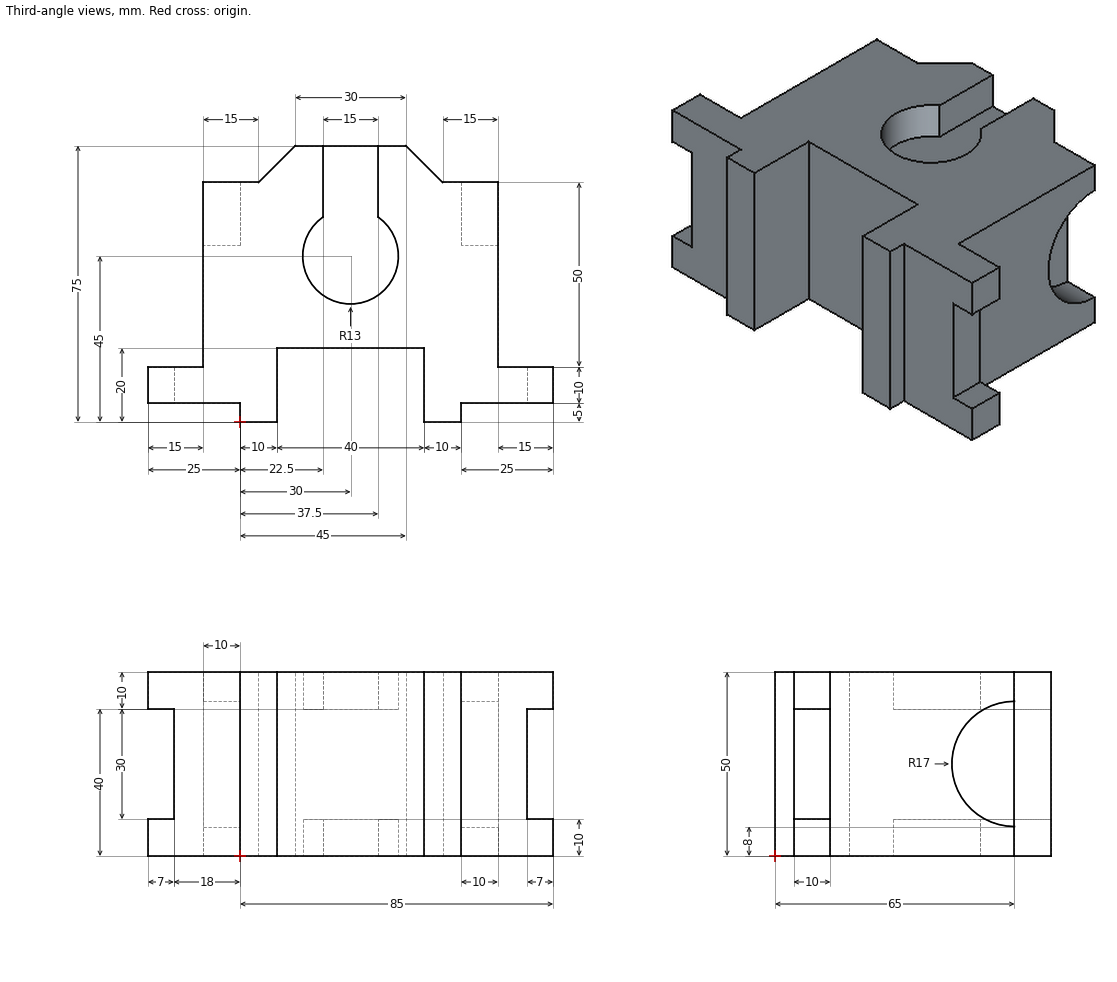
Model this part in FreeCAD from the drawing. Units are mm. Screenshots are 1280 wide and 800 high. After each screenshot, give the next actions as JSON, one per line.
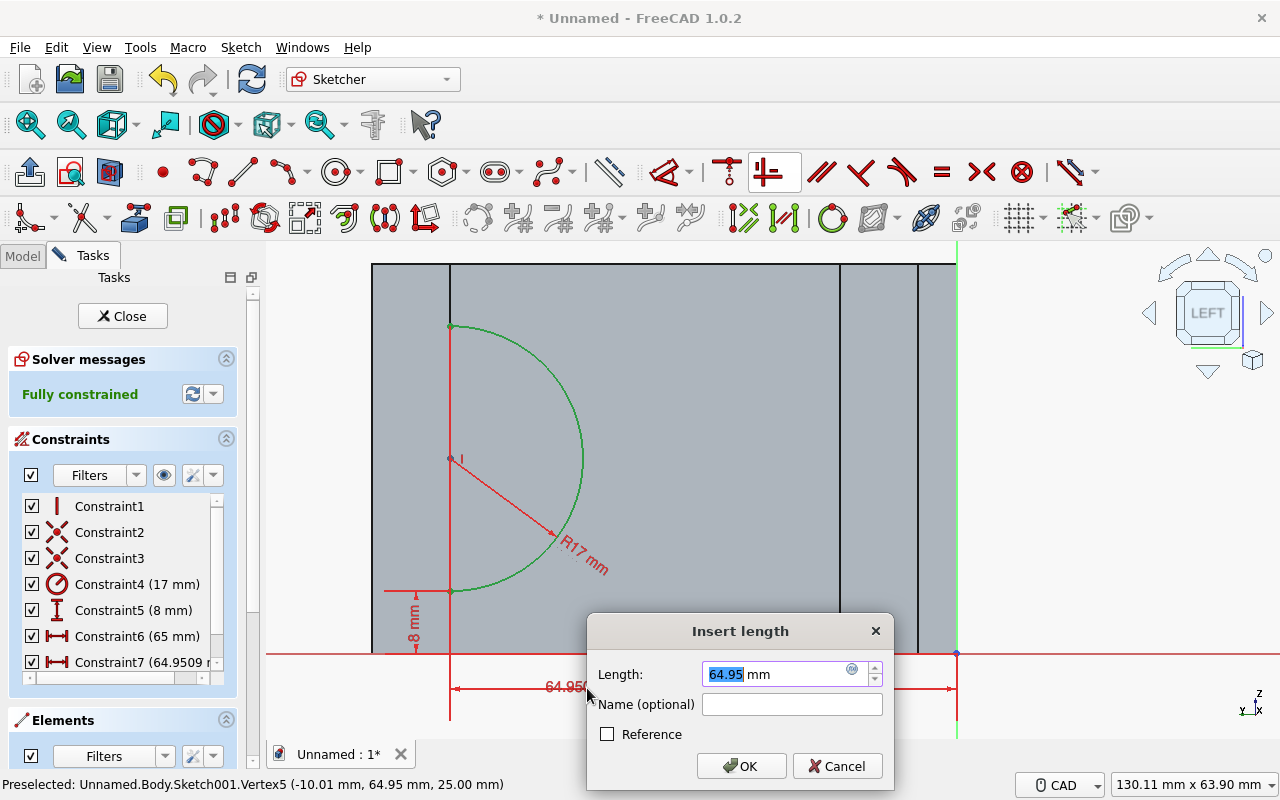
{"action": "type", "text": "65"}
{"action": "key", "text": "Return"}
{"action": "key", "text": "Escape"}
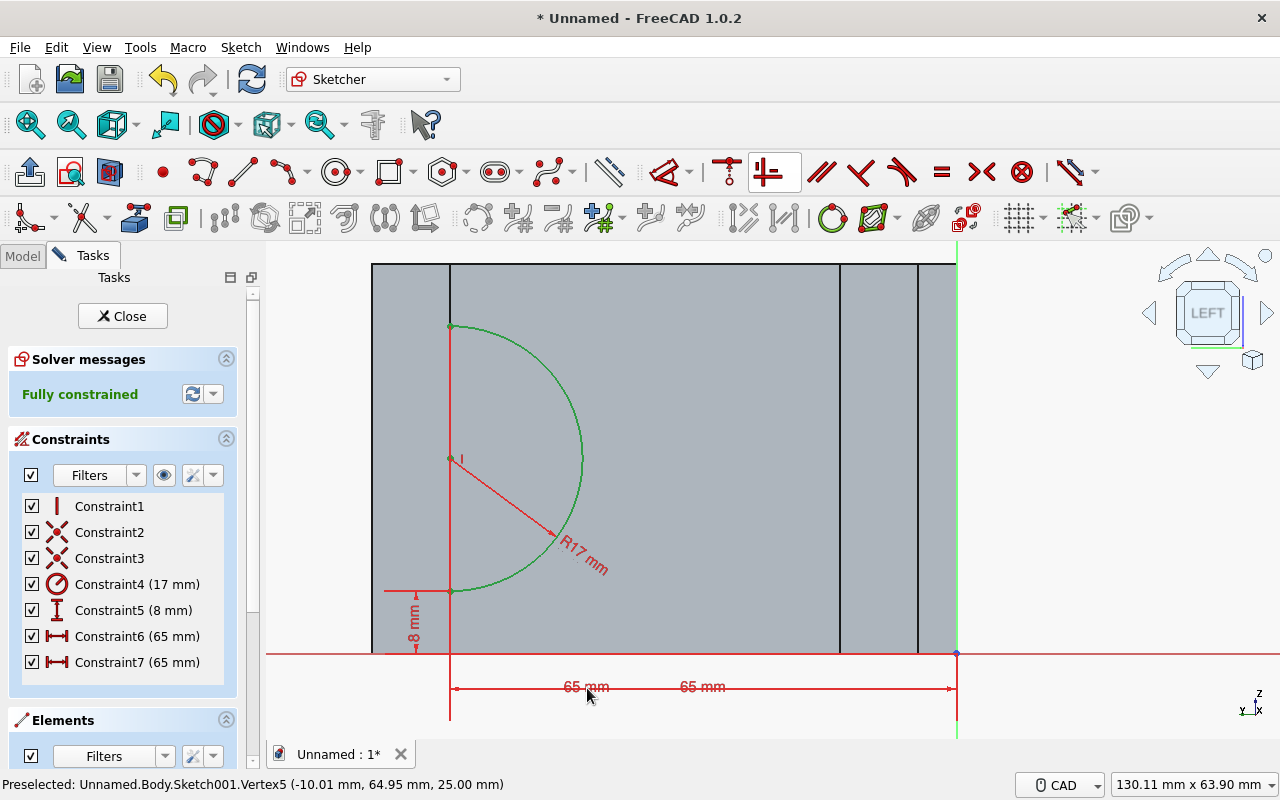
{"action": "left_click", "coordinate": [123, 316]}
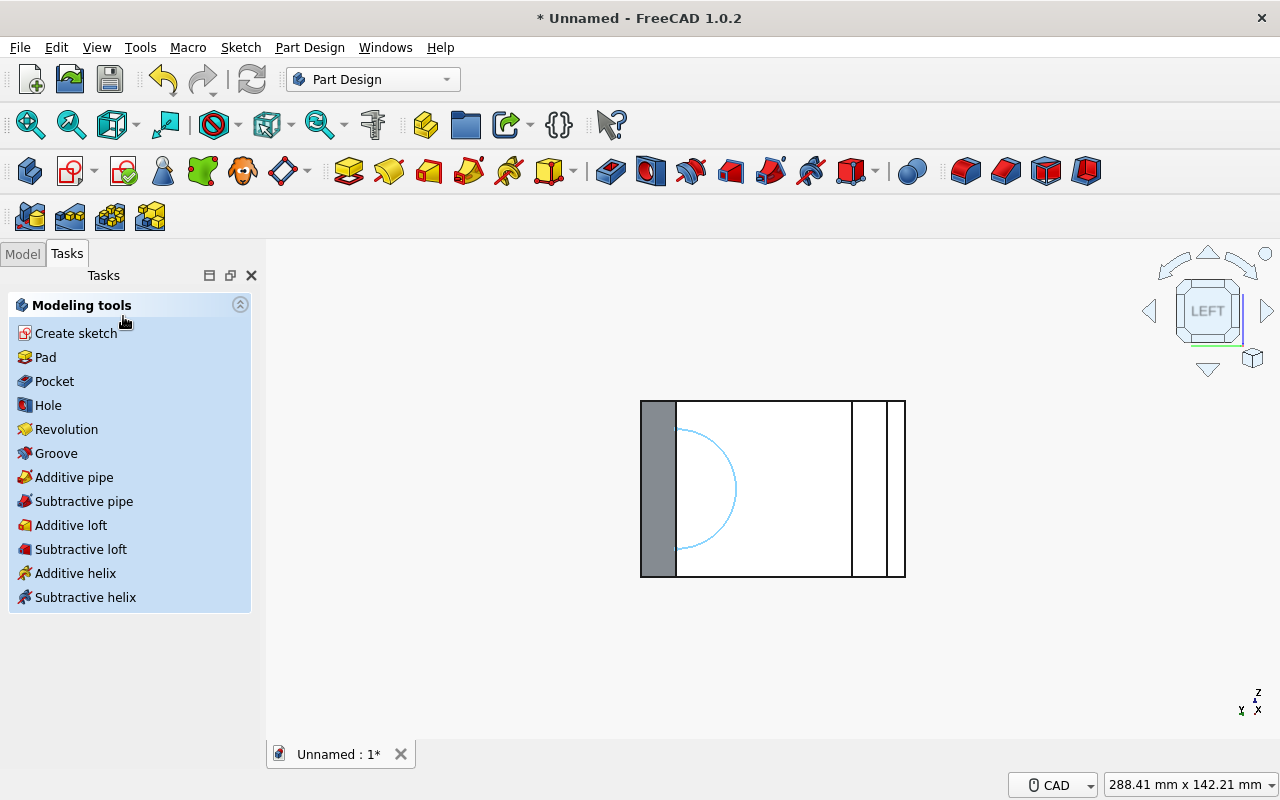
{"action": "left_click", "coordinate": [612, 172]}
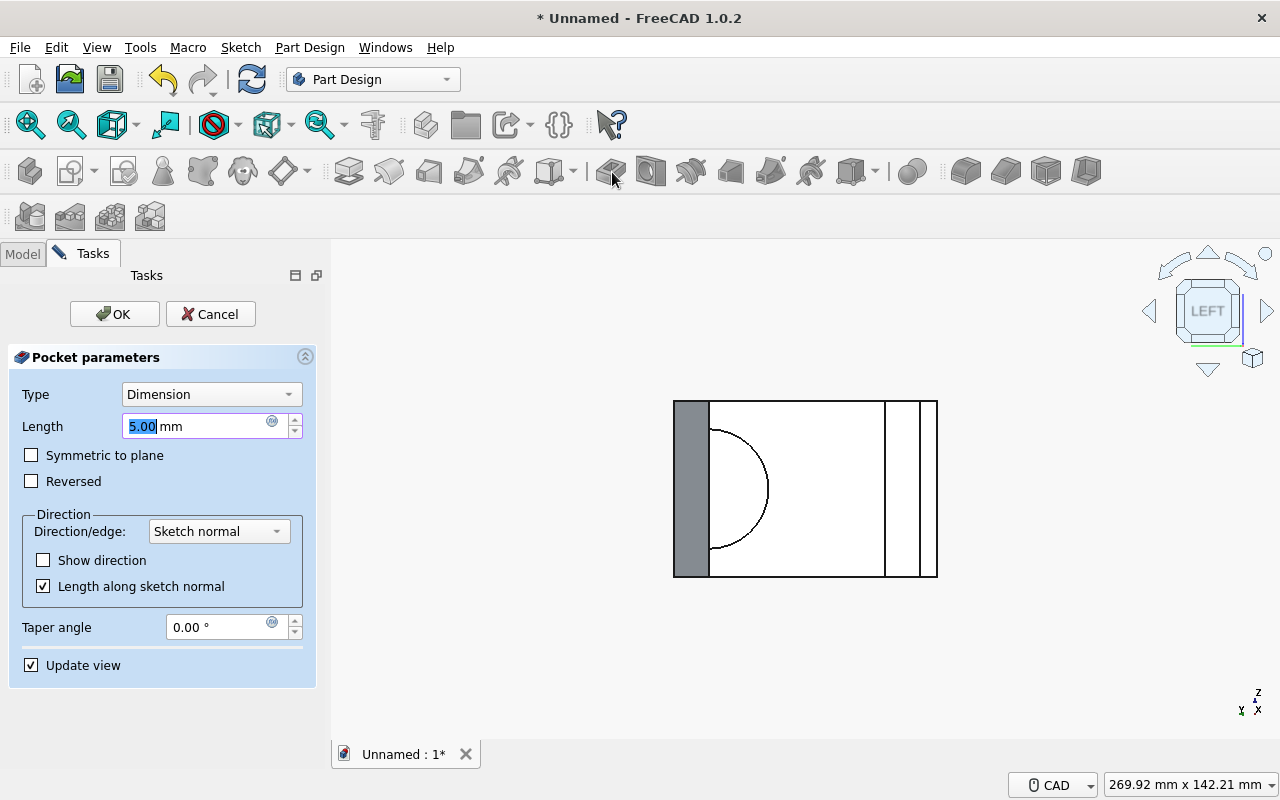
{"action": "type", "text": "10"}
{"action": "key", "text": "Tab"}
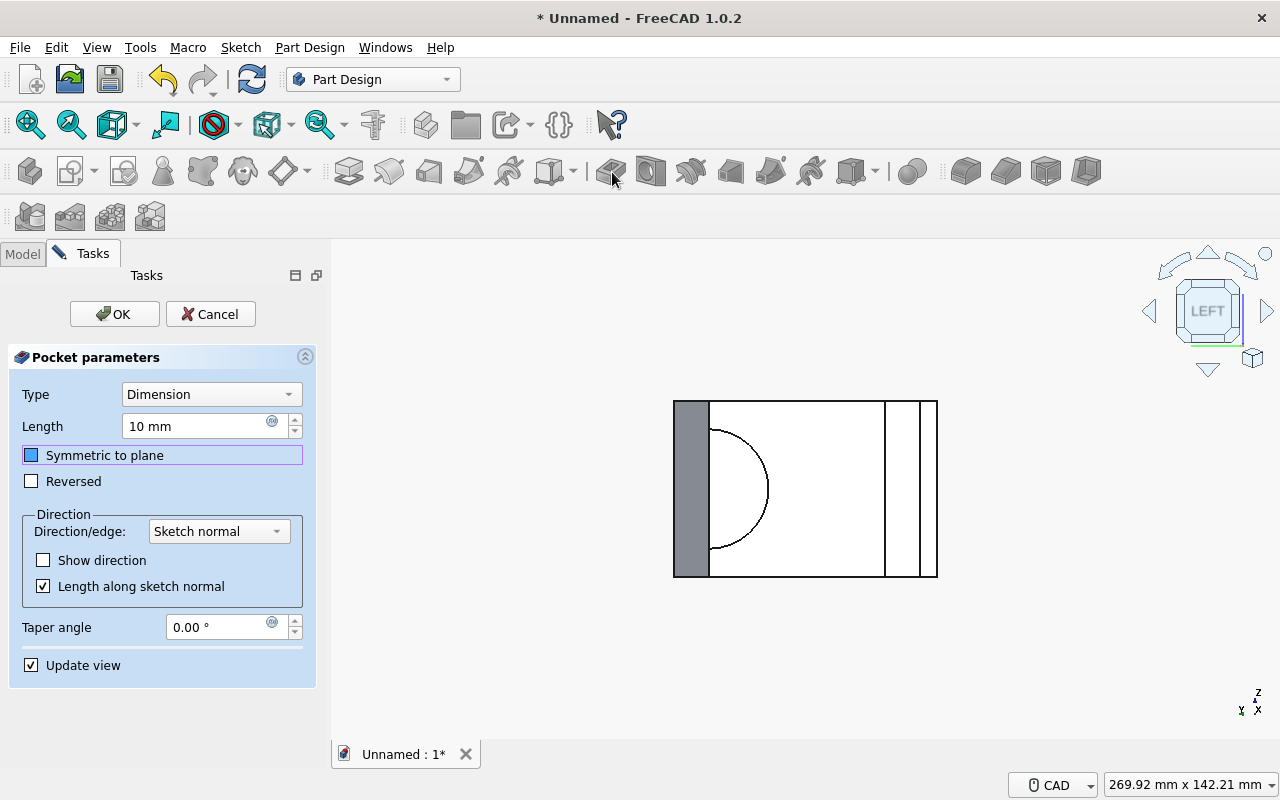
{"action": "left_click", "coordinate": [115, 314]}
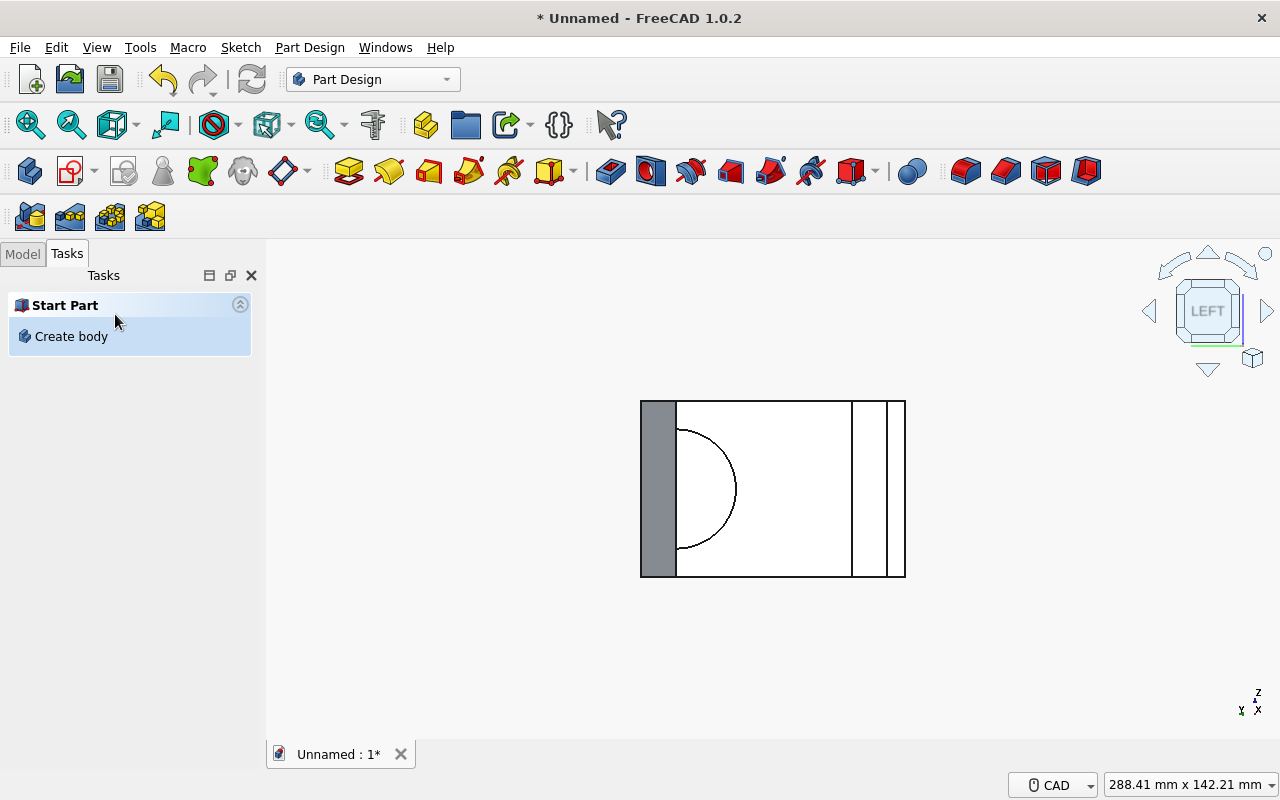
{"action": "left_click", "coordinate": [32, 126]}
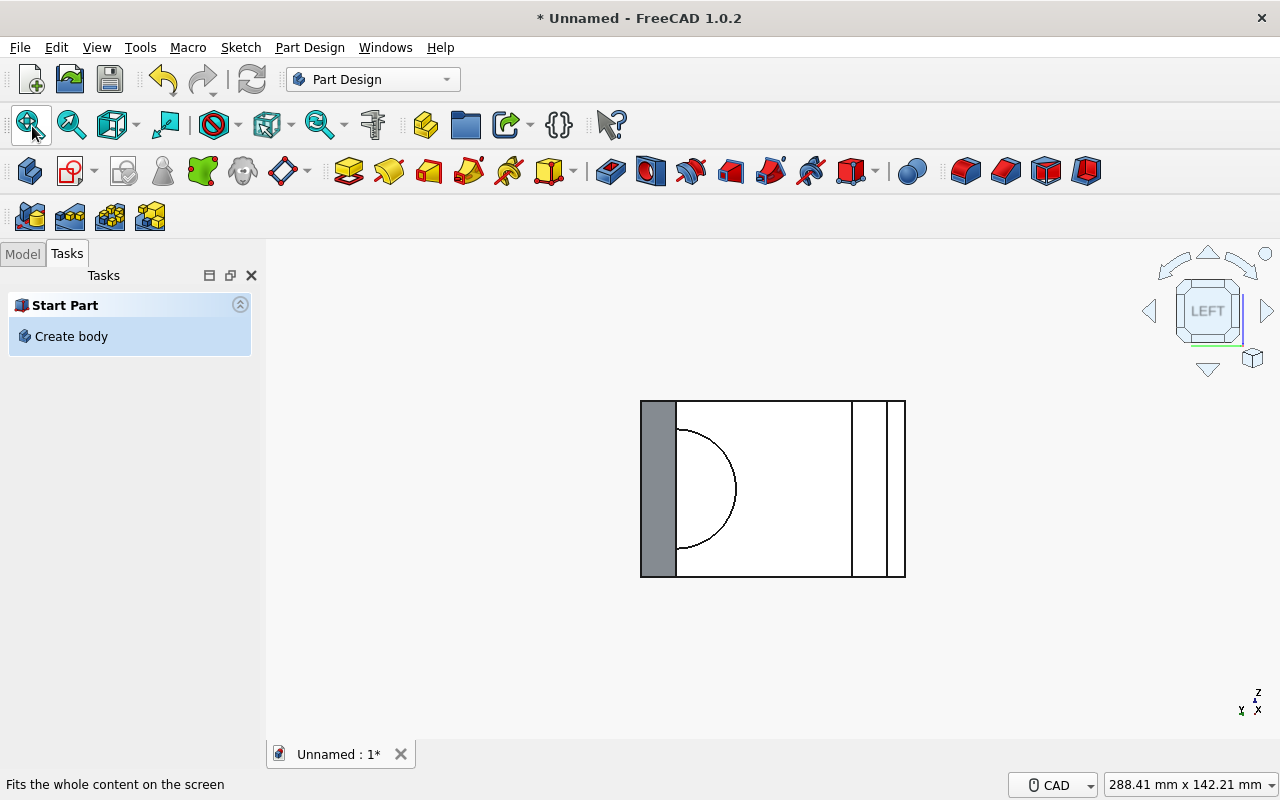
{"action": "key", "text": "0"}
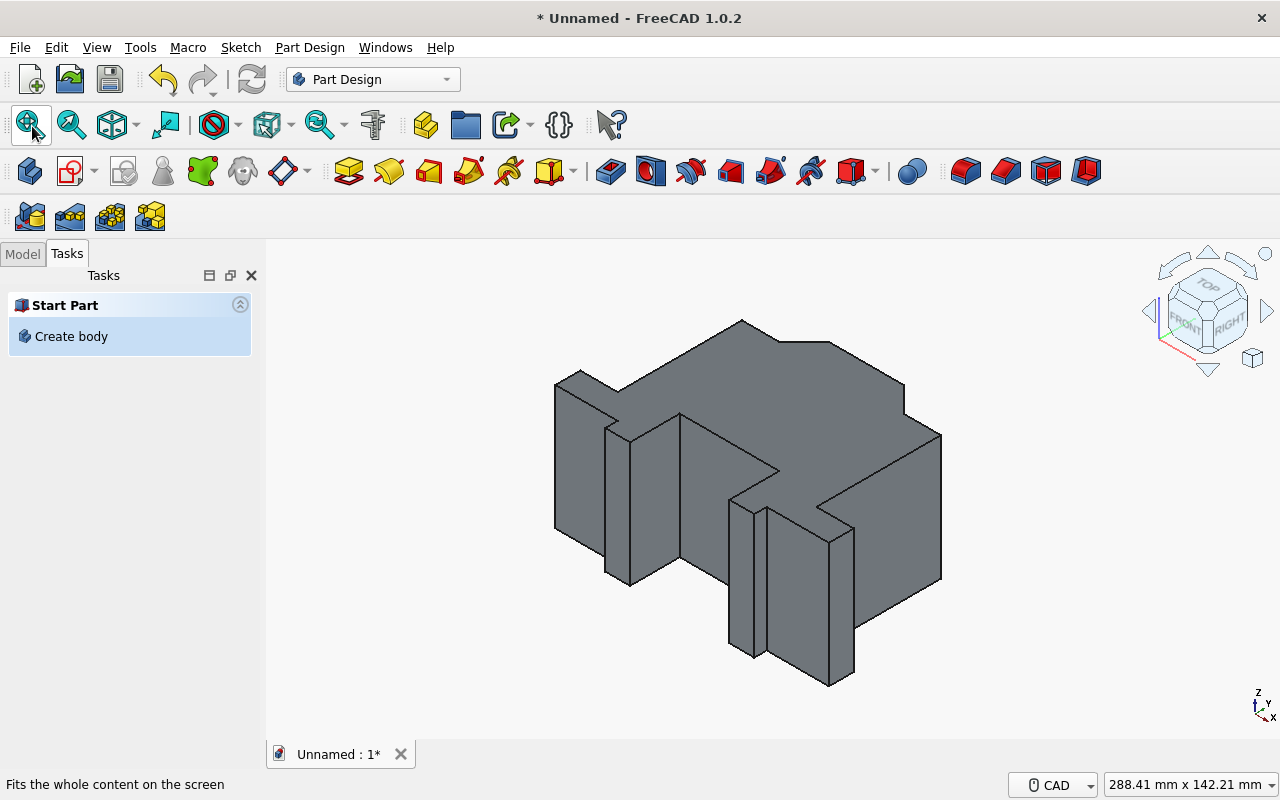
{"action": "key", "text": "3"}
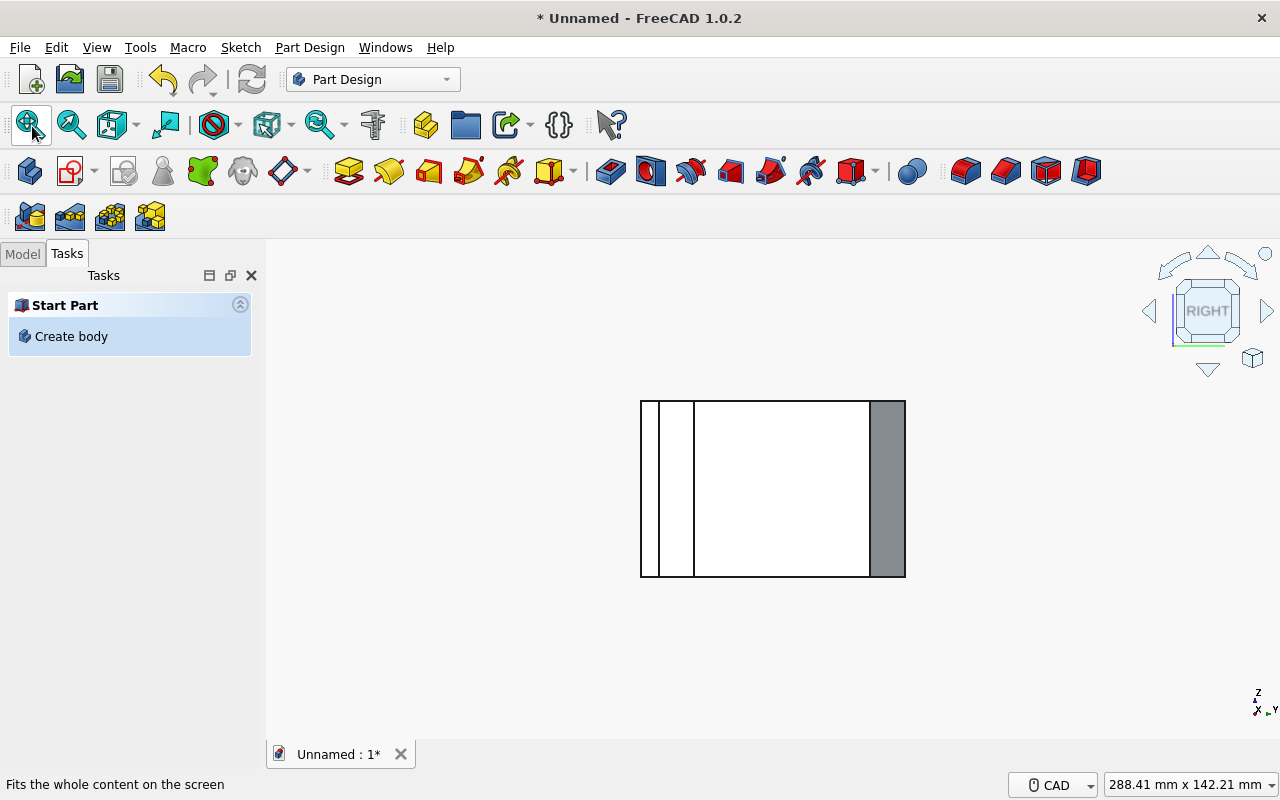
{"action": "key", "text": "v f"}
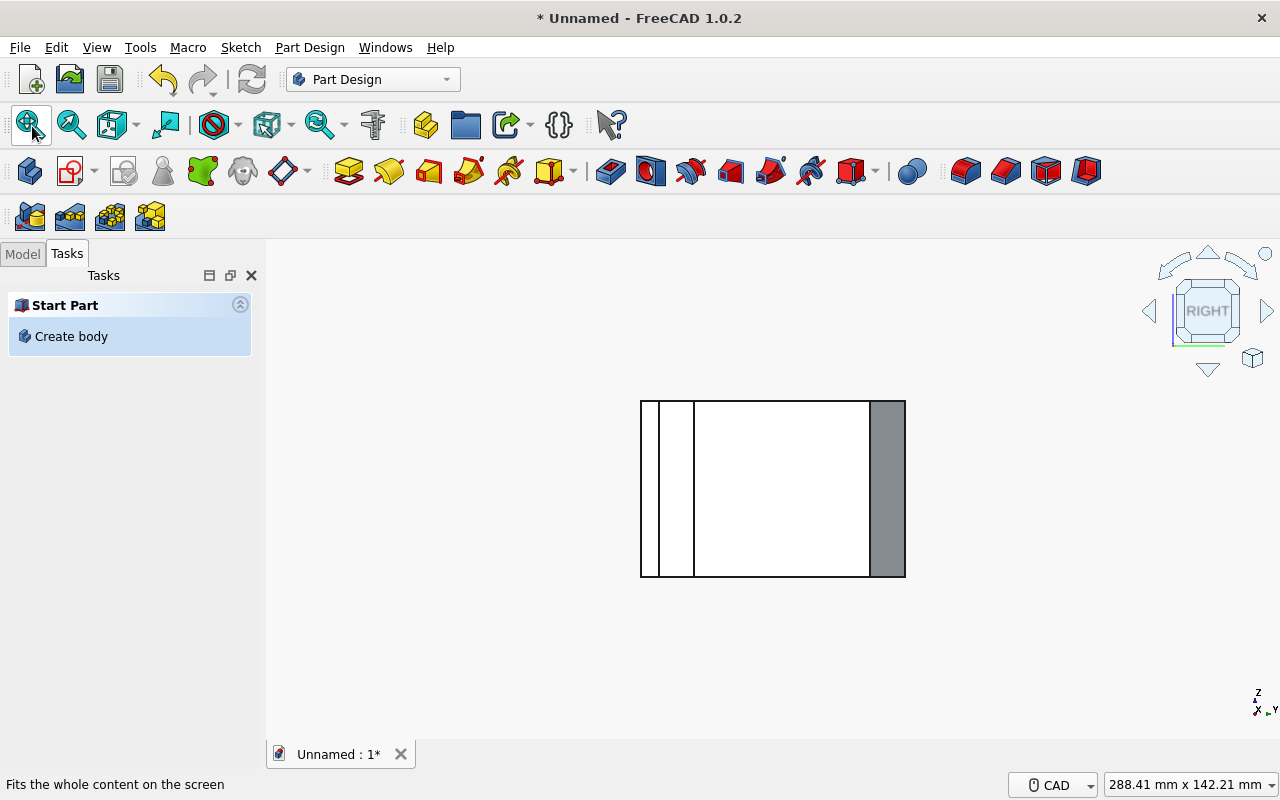
{"action": "left_click", "coordinate": [650, 413]}